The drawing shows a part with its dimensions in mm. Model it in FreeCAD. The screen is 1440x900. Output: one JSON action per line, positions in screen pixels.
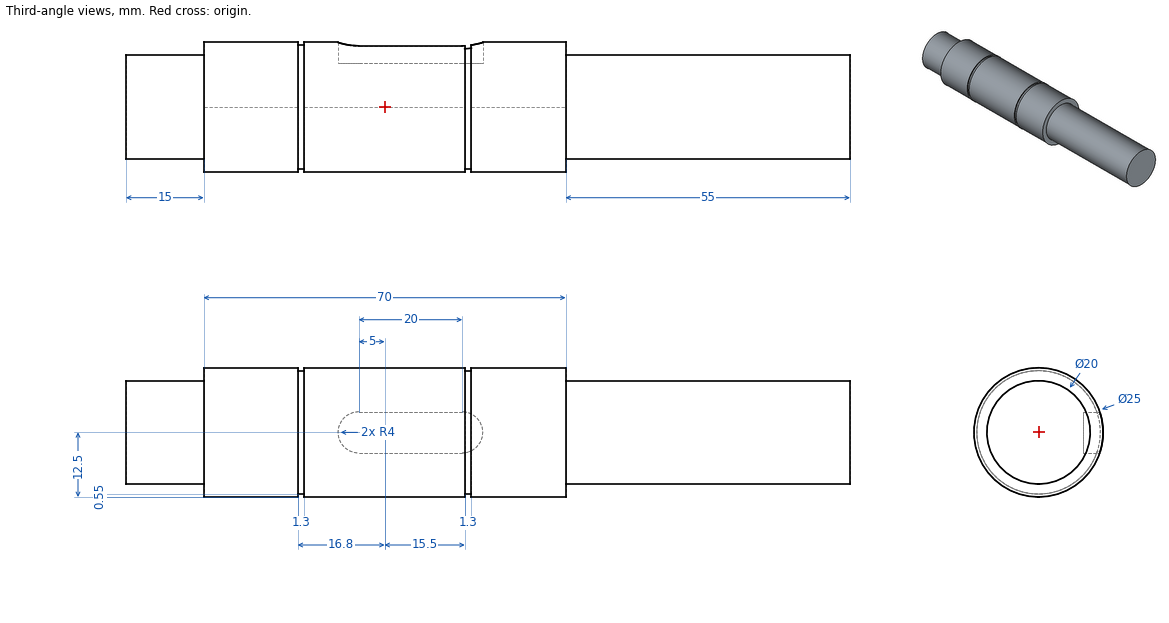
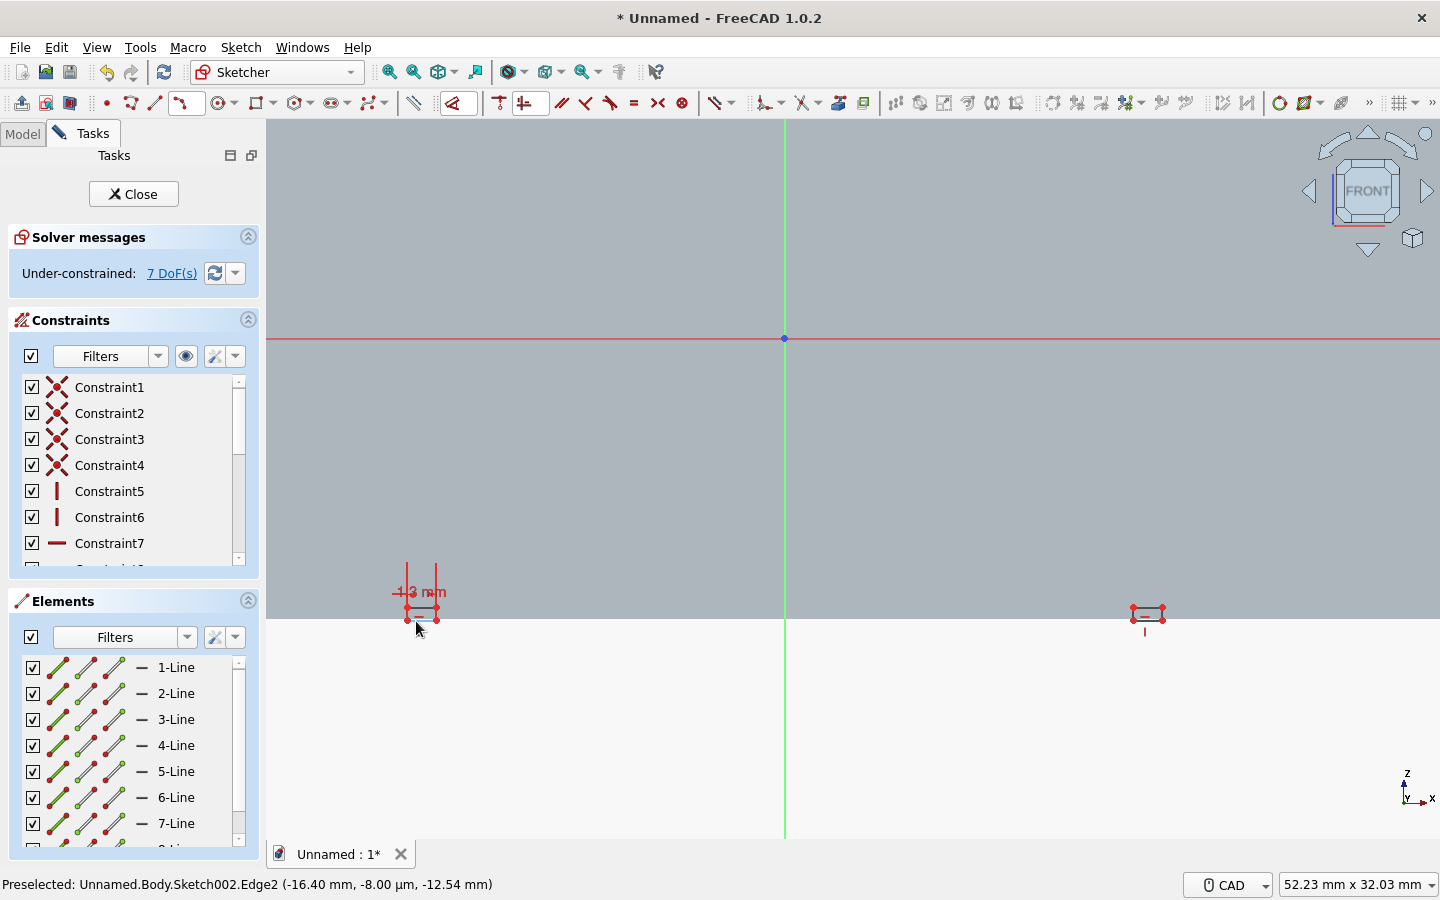
{"action": "scroll", "coordinate": [1142, 621], "scroll_direction": "up", "scroll_amount": 3}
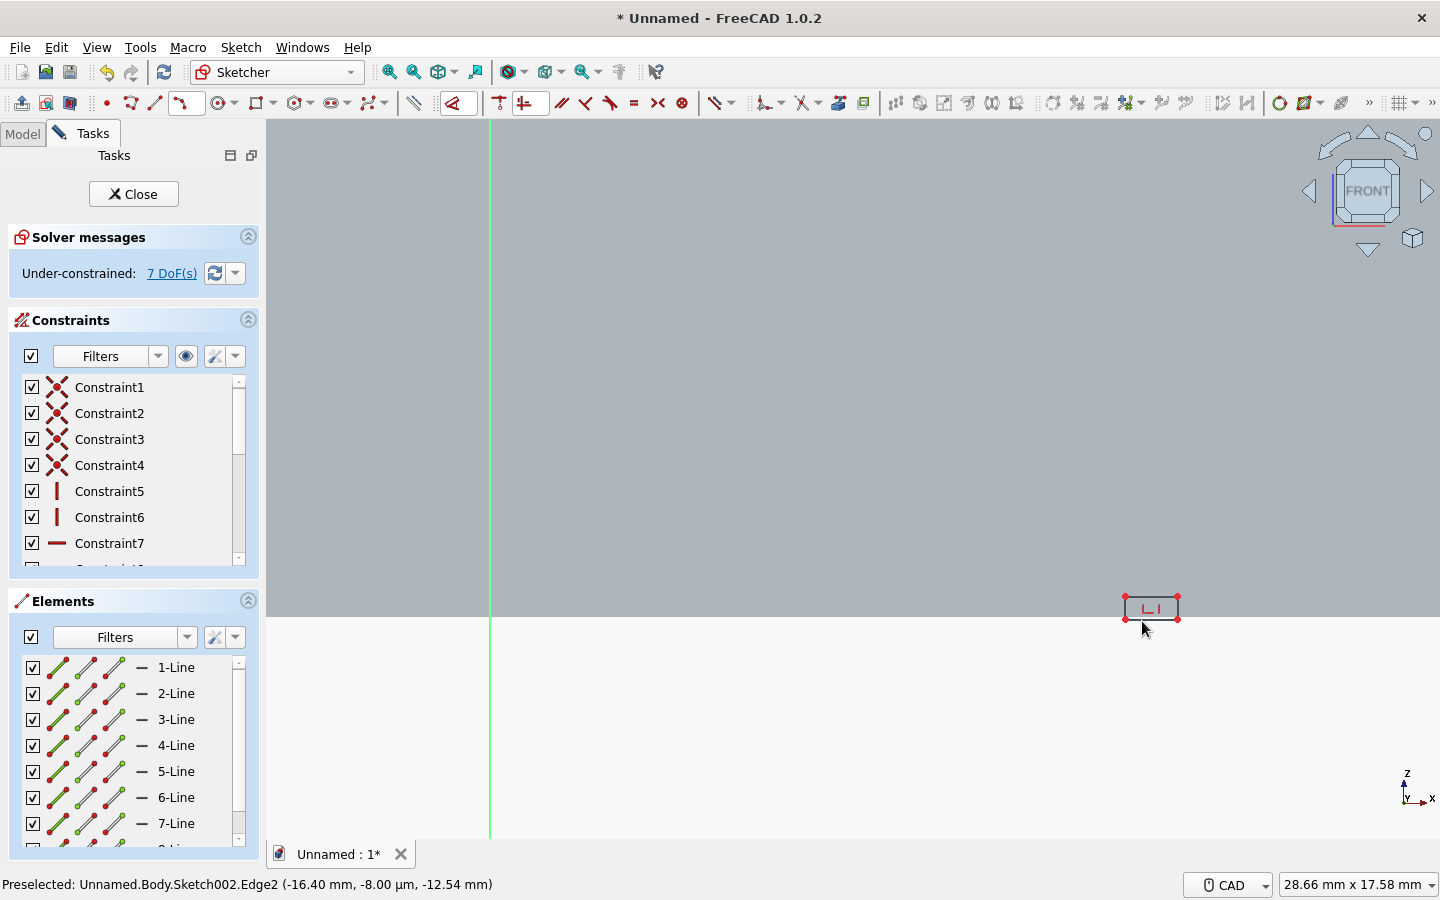
{"action": "left_click", "coordinate": [1141, 620]}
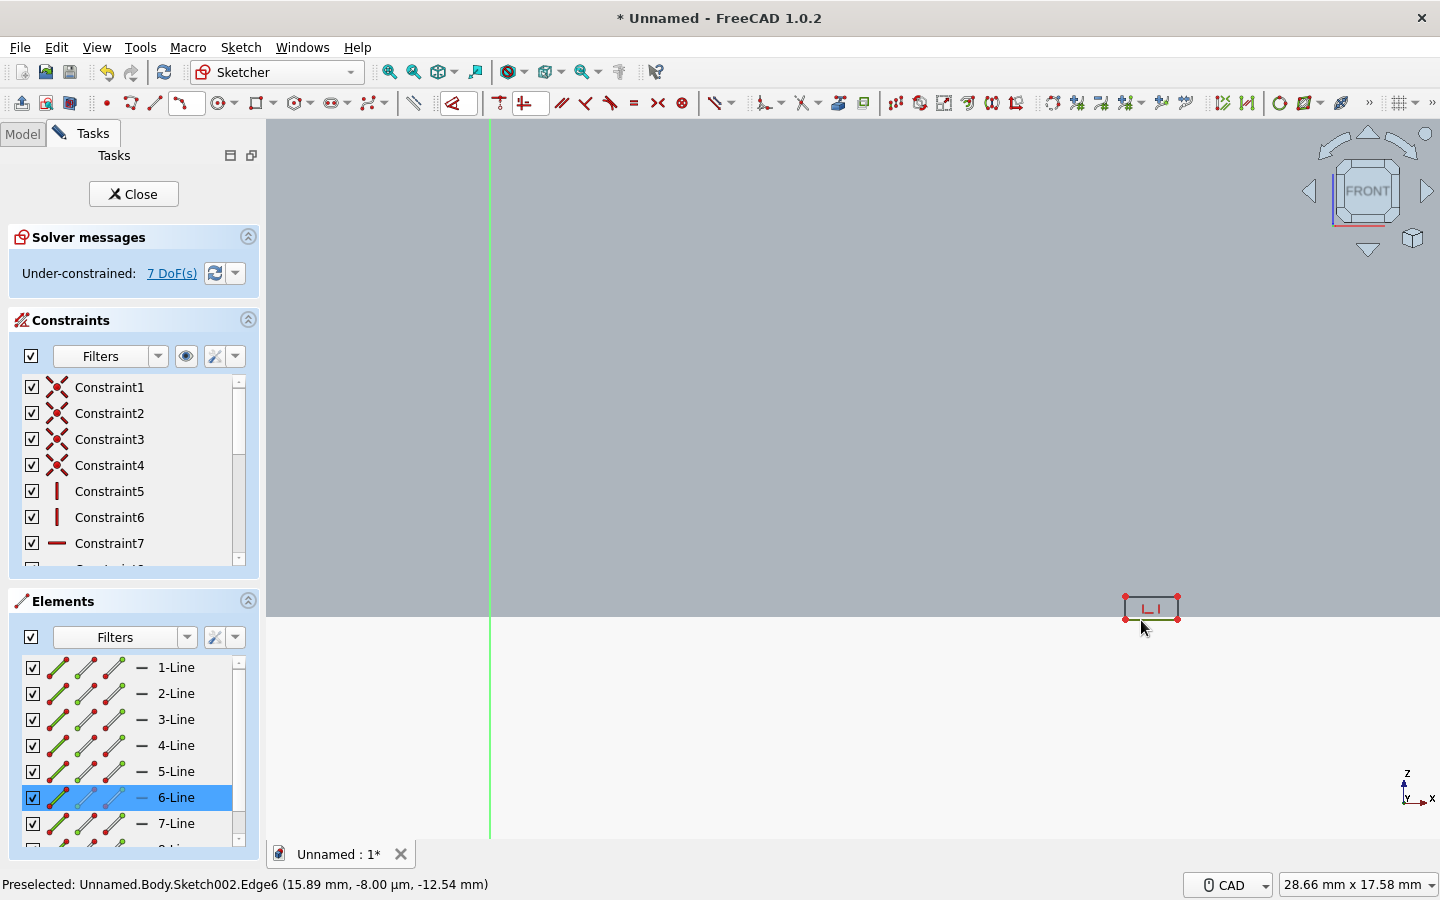
{"action": "key", "text": "l"}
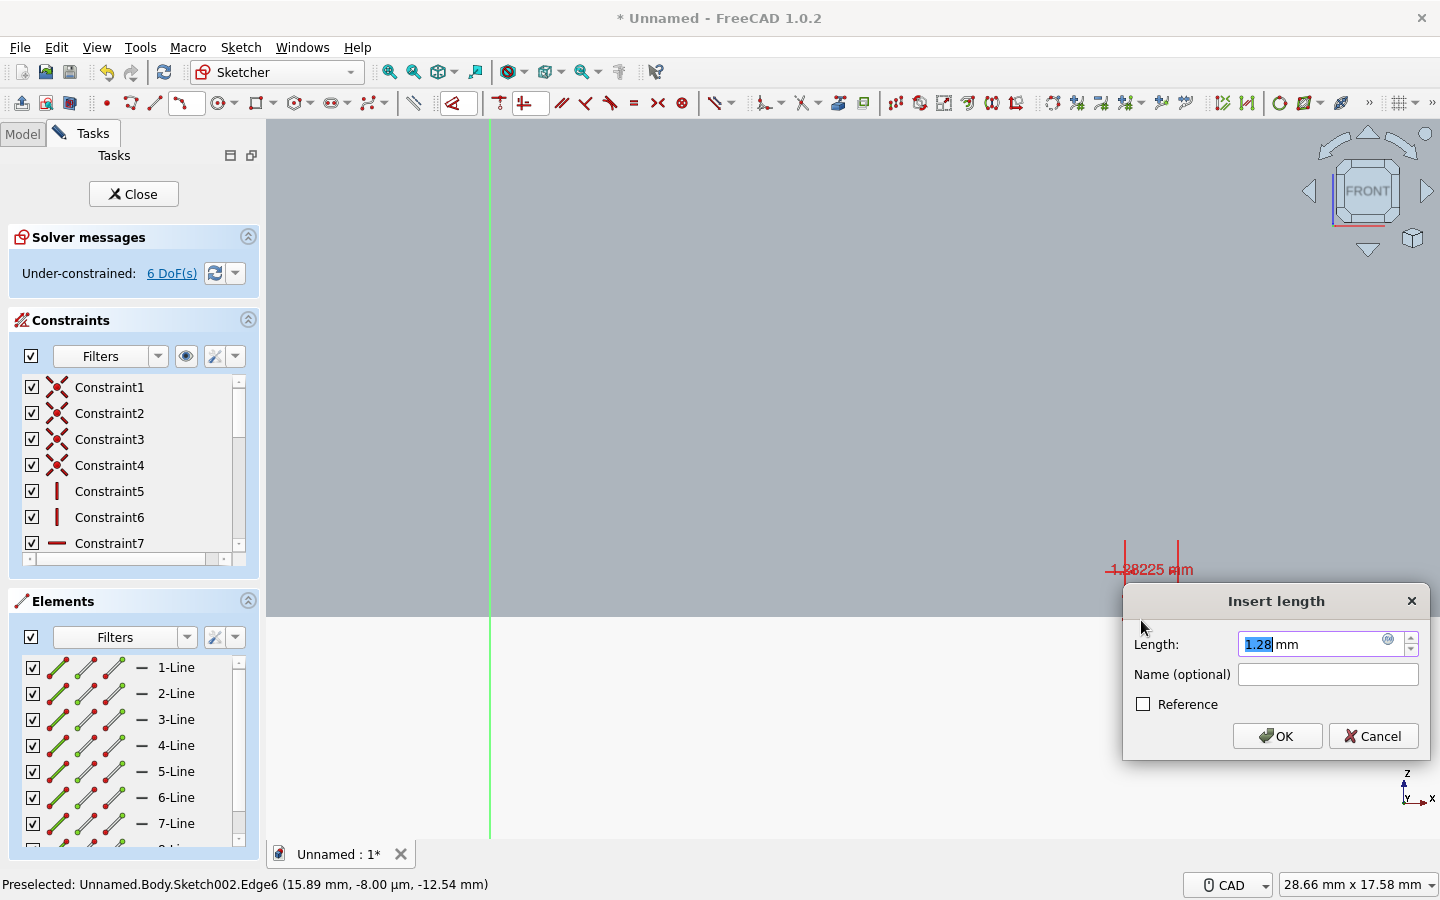
{"action": "type", "text": "1.3"}
{"action": "key", "text": "Return"}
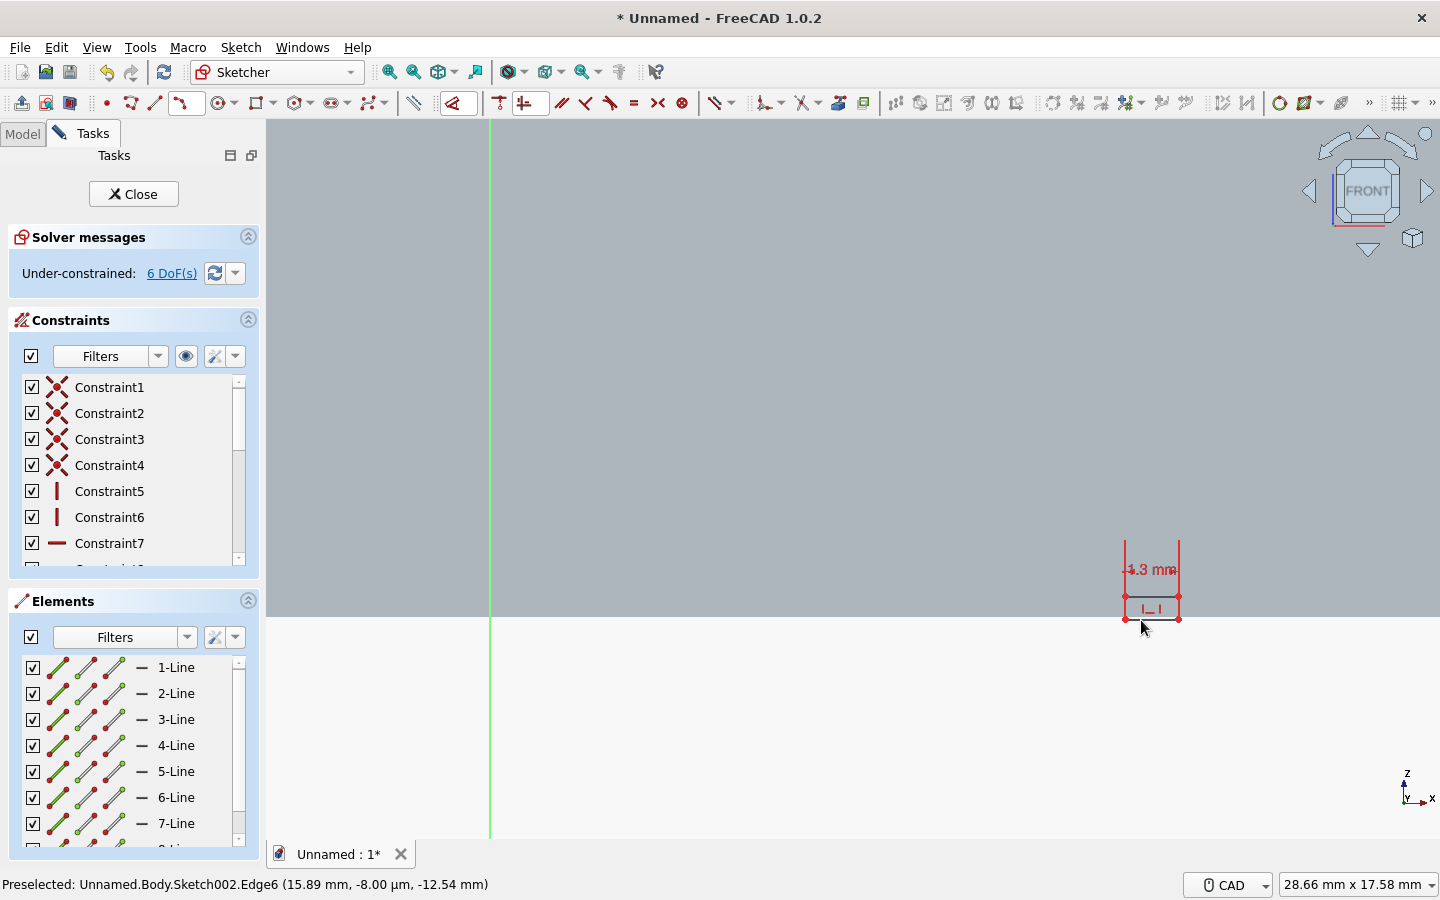
{"action": "scroll", "coordinate": [1142, 621], "scroll_direction": "down", "scroll_amount": 3}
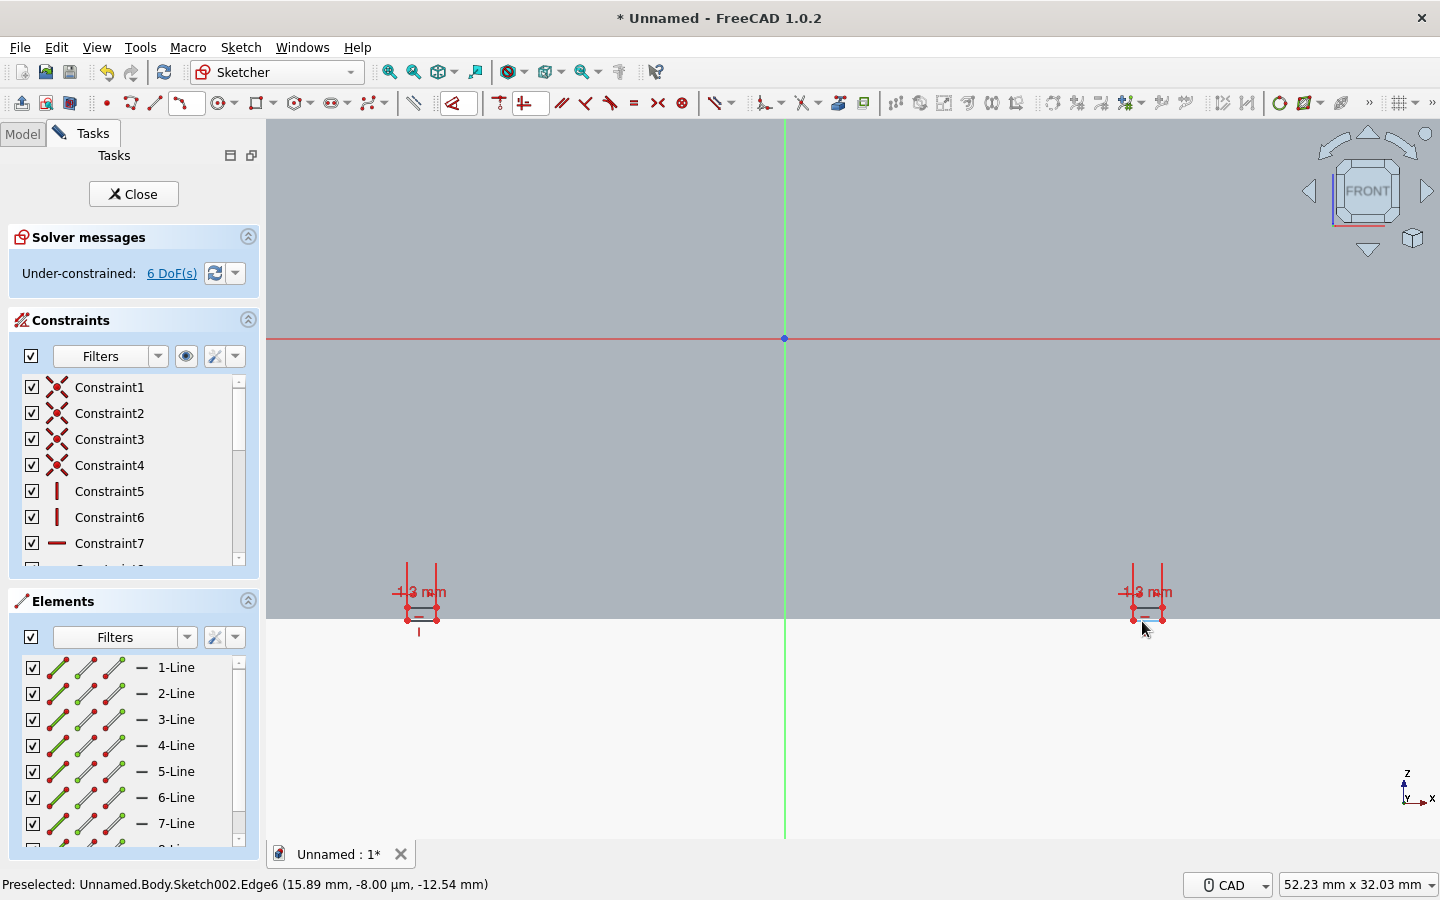
{"action": "scroll", "coordinate": [407, 613], "scroll_direction": "up", "scroll_amount": 6}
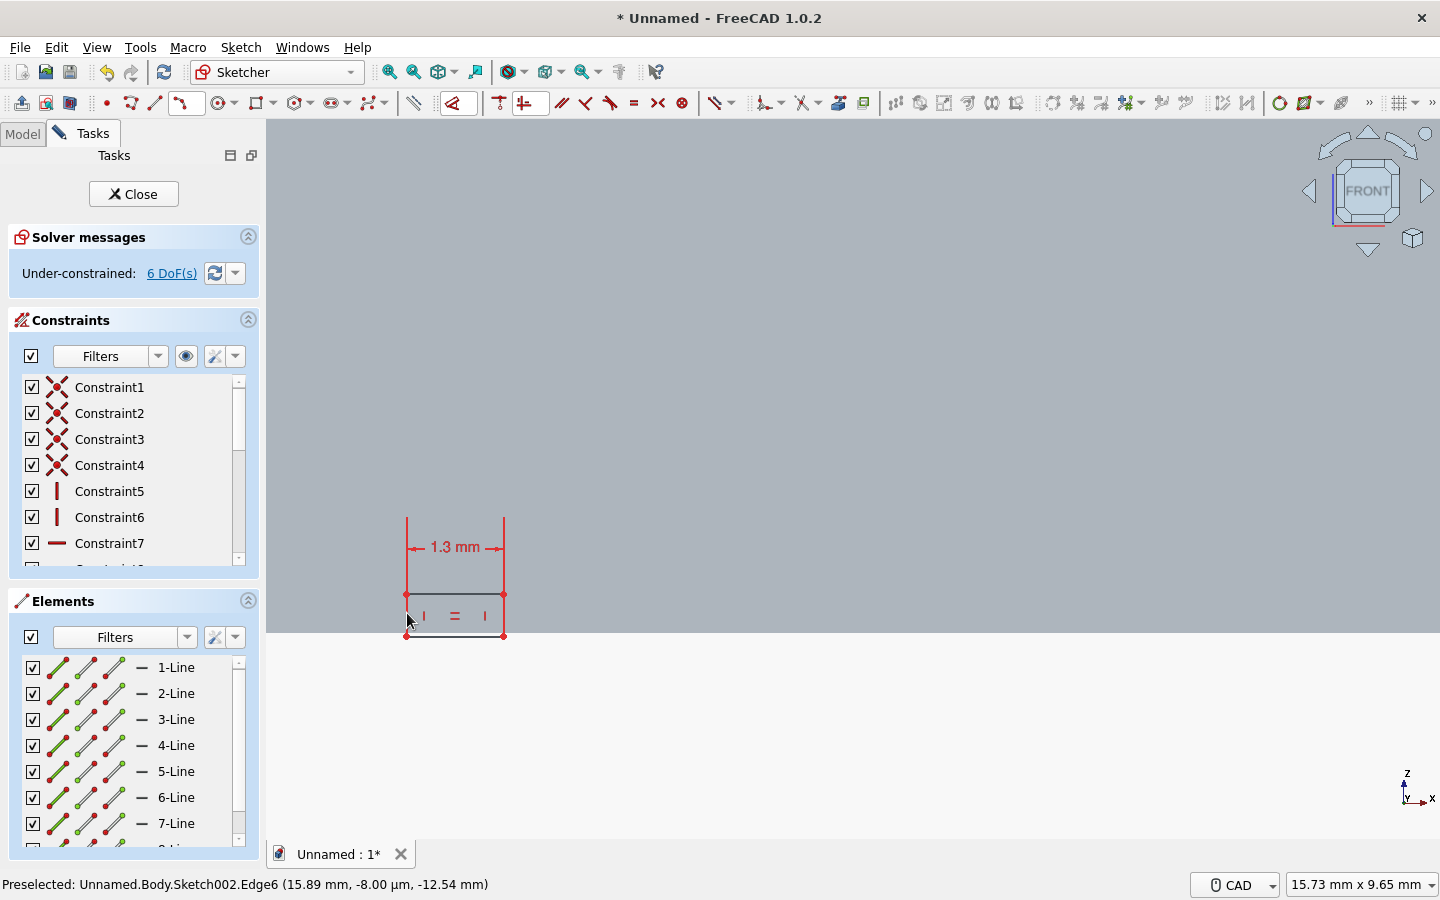
{"action": "left_click", "coordinate": [407, 611]}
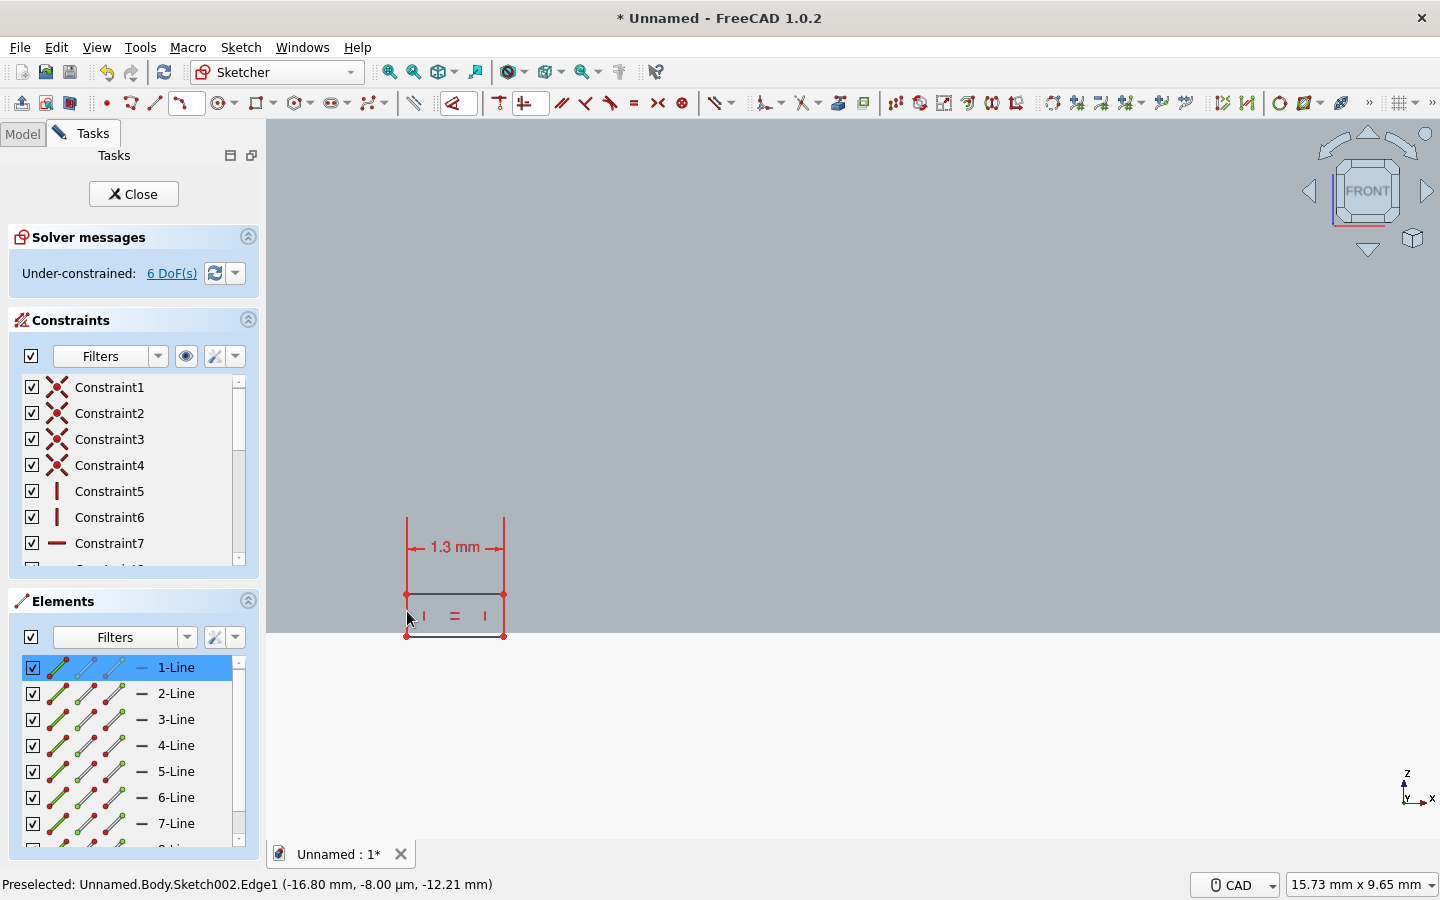
{"action": "key", "text": "i"}